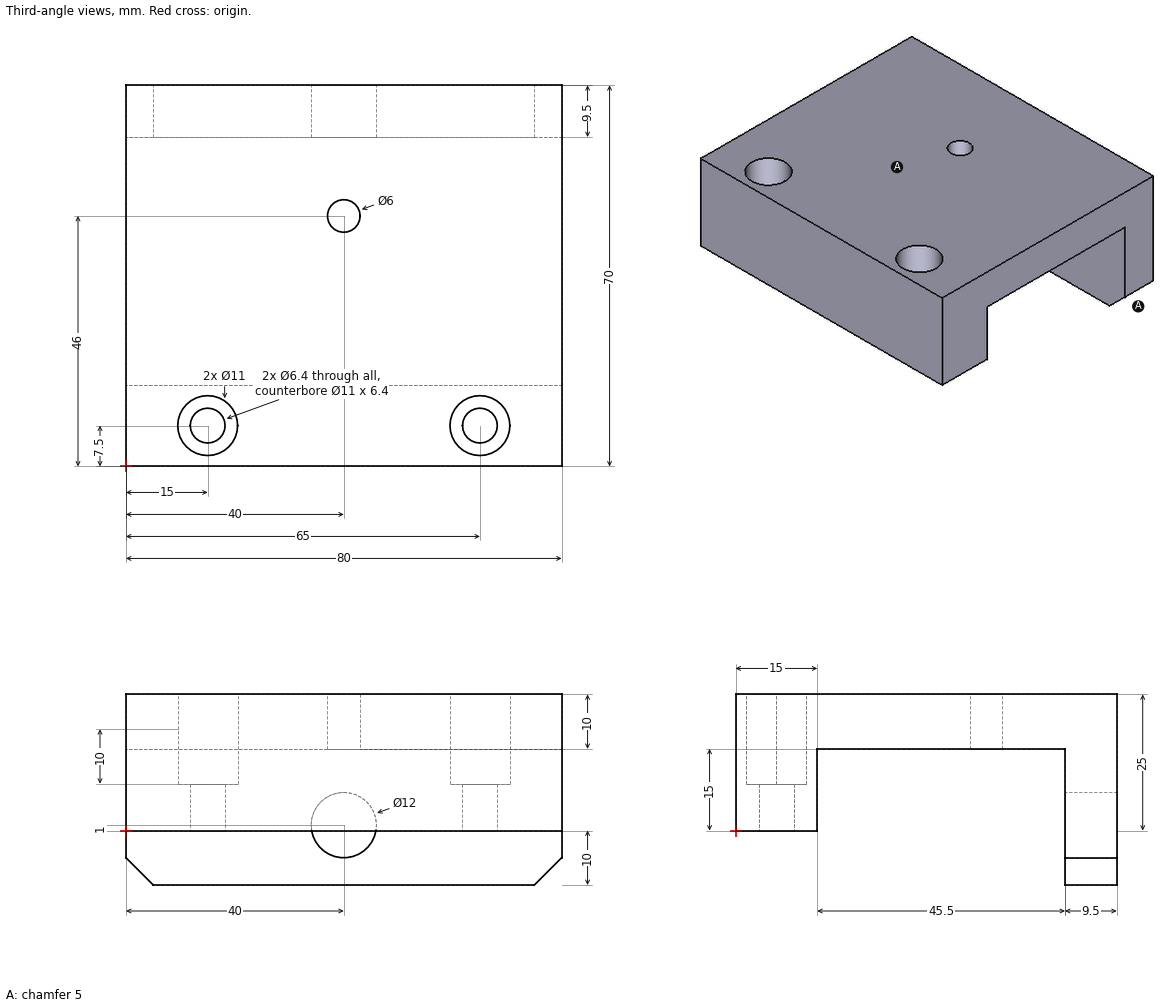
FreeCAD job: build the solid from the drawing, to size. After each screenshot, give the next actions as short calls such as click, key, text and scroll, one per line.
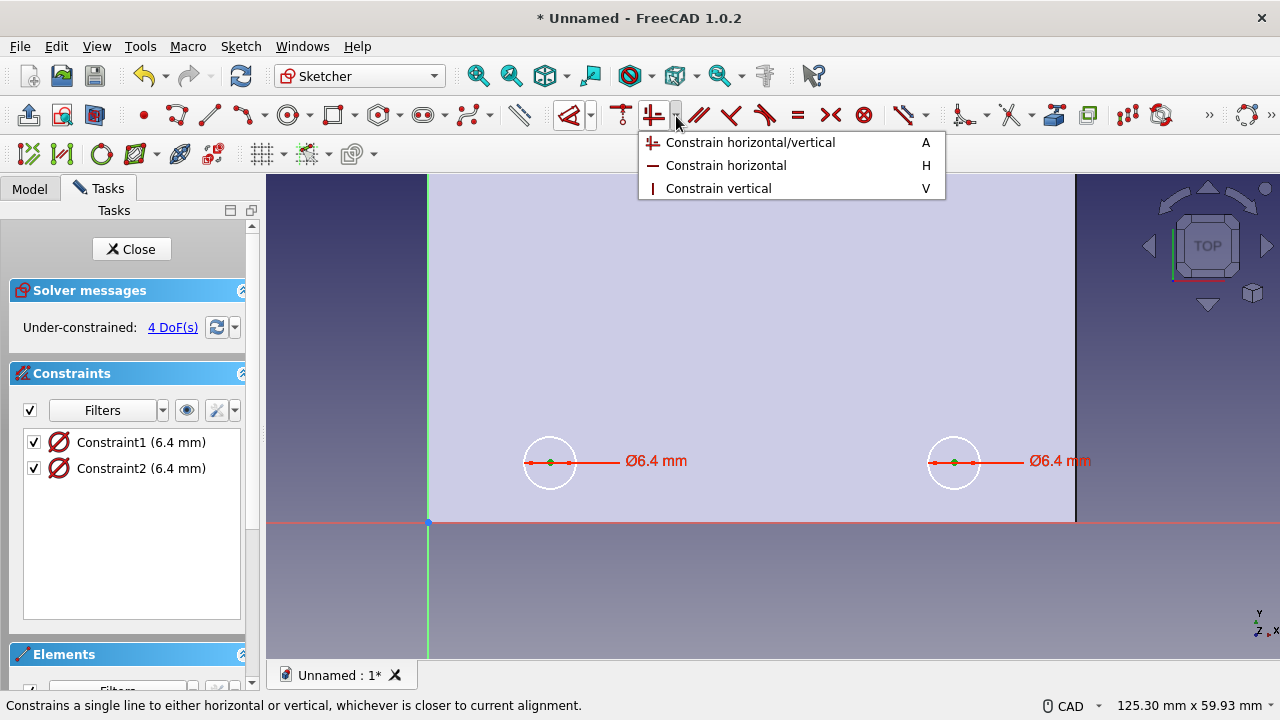
click(792, 166)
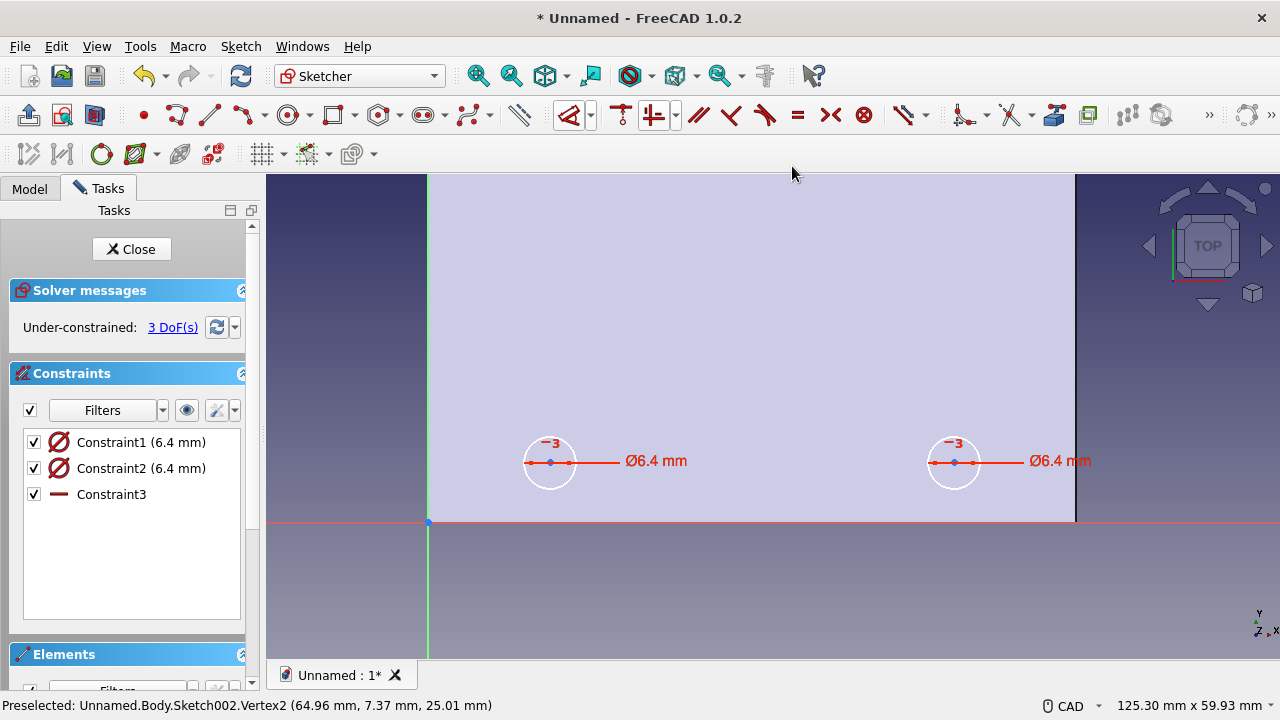
click(550, 463)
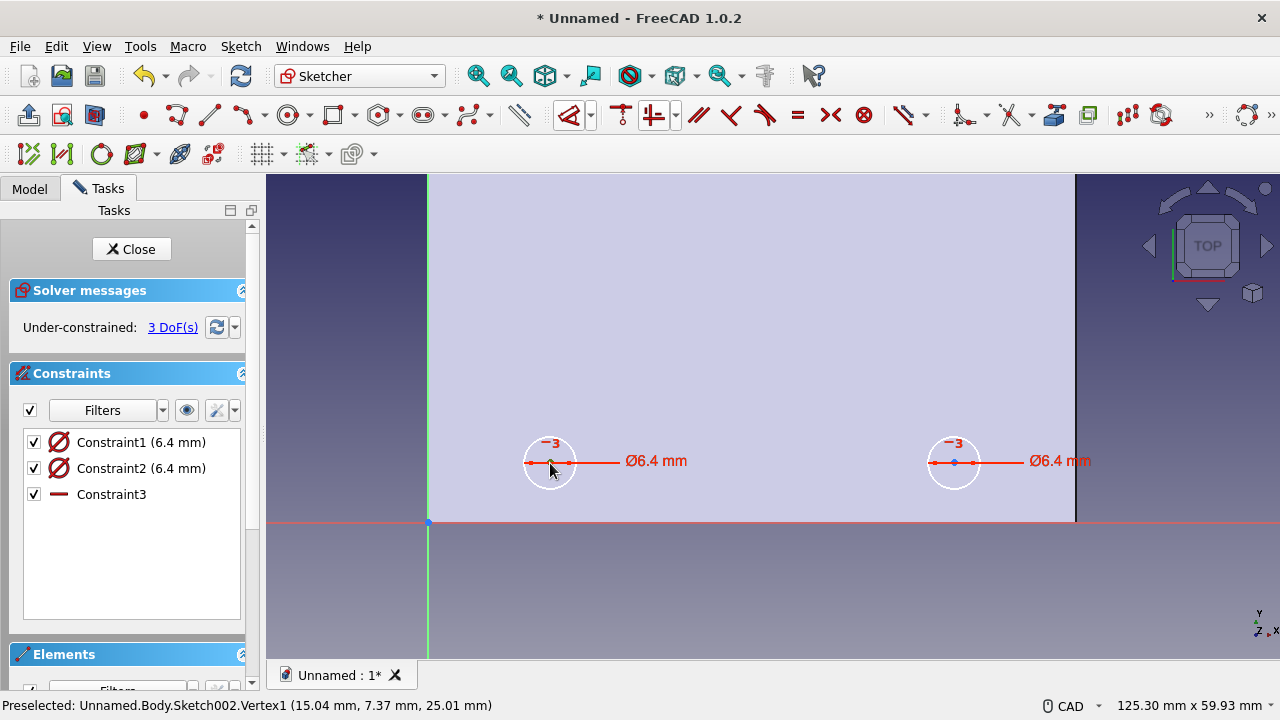
click(590, 116)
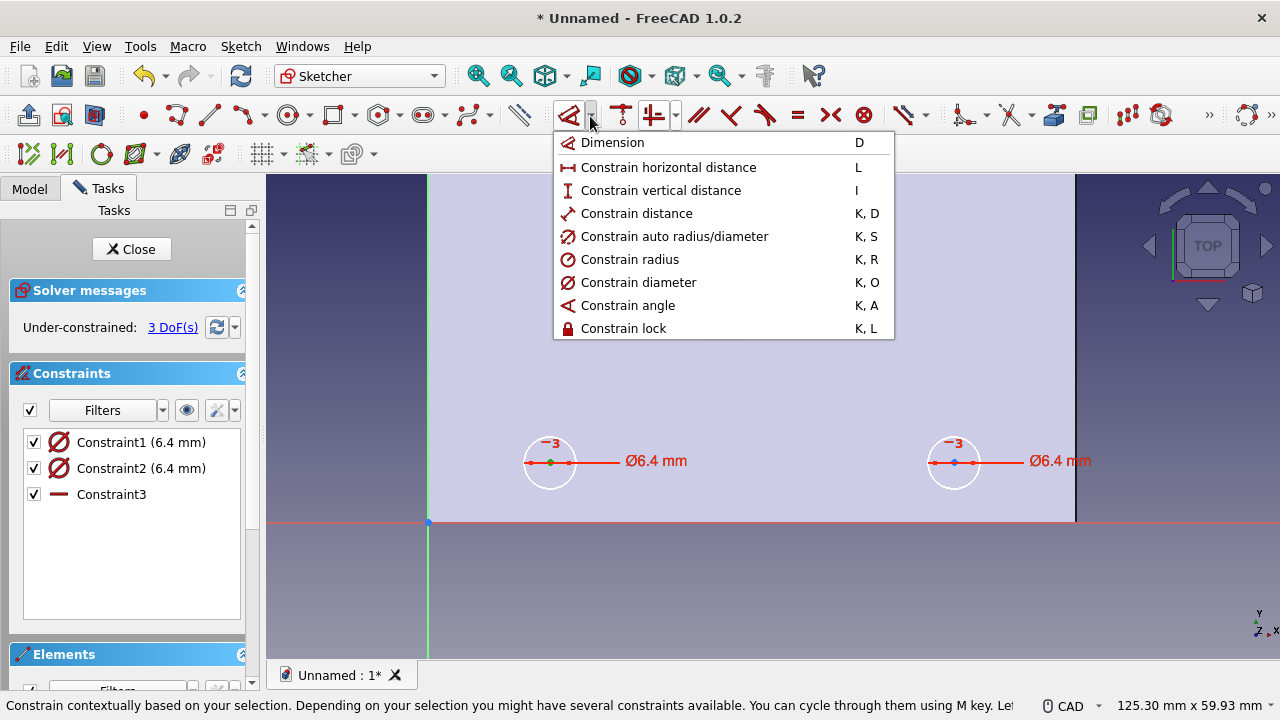
click(724, 168)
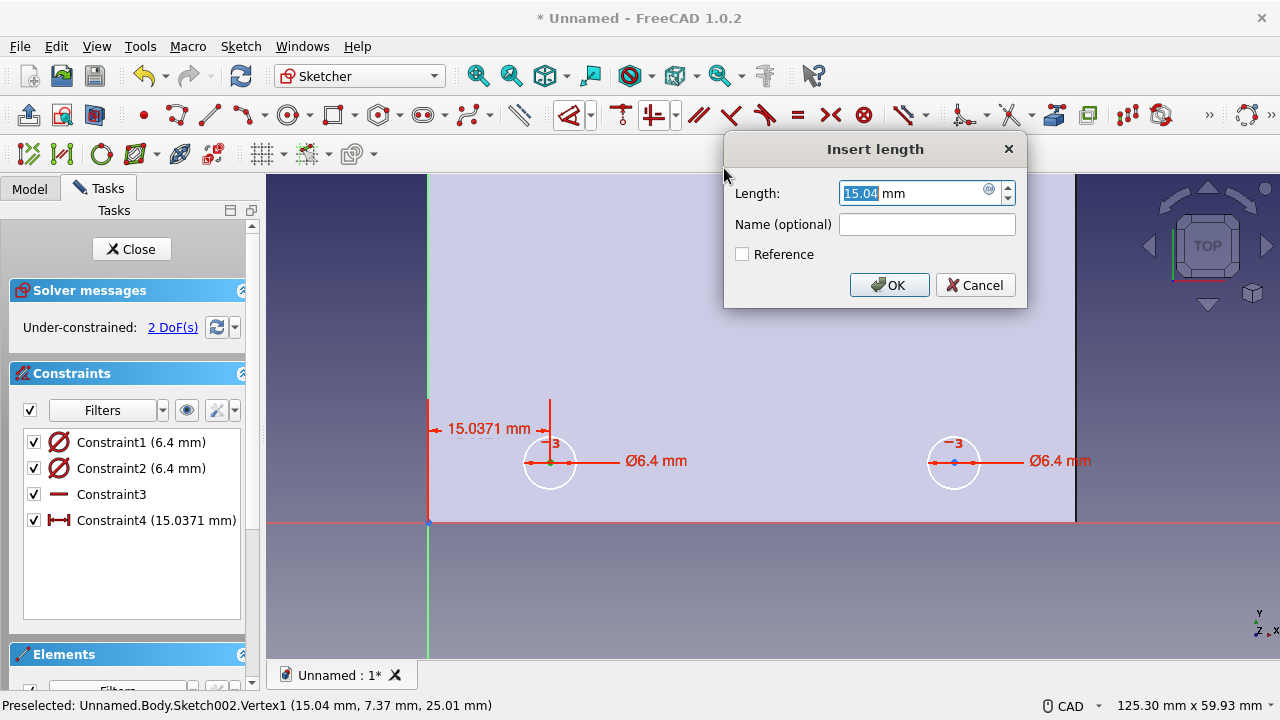
text(15)
key(Return)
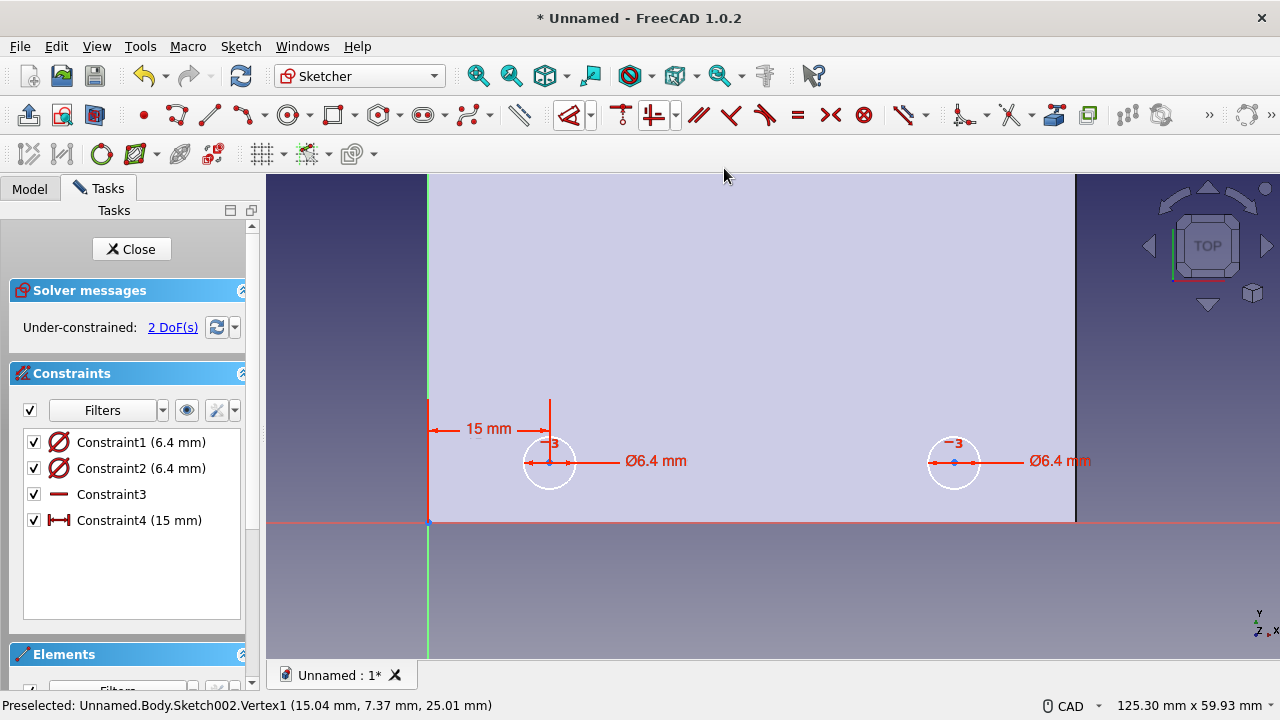
click(954, 463)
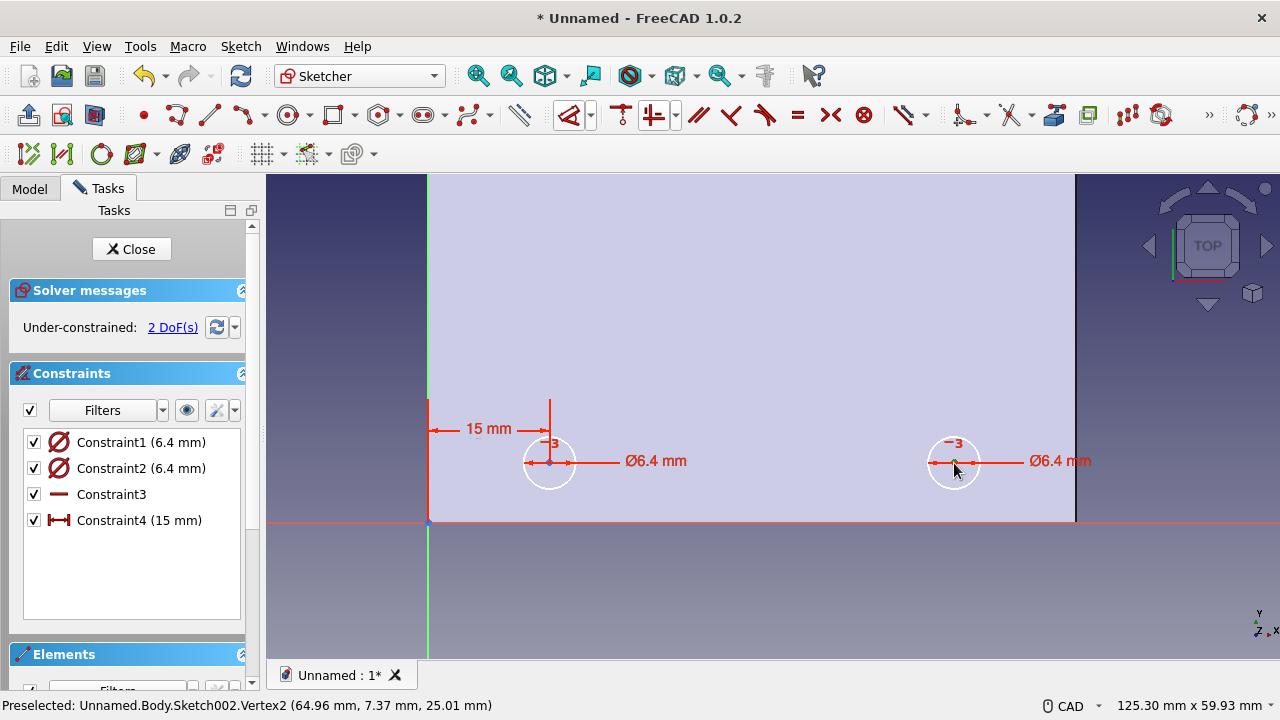
click(590, 116)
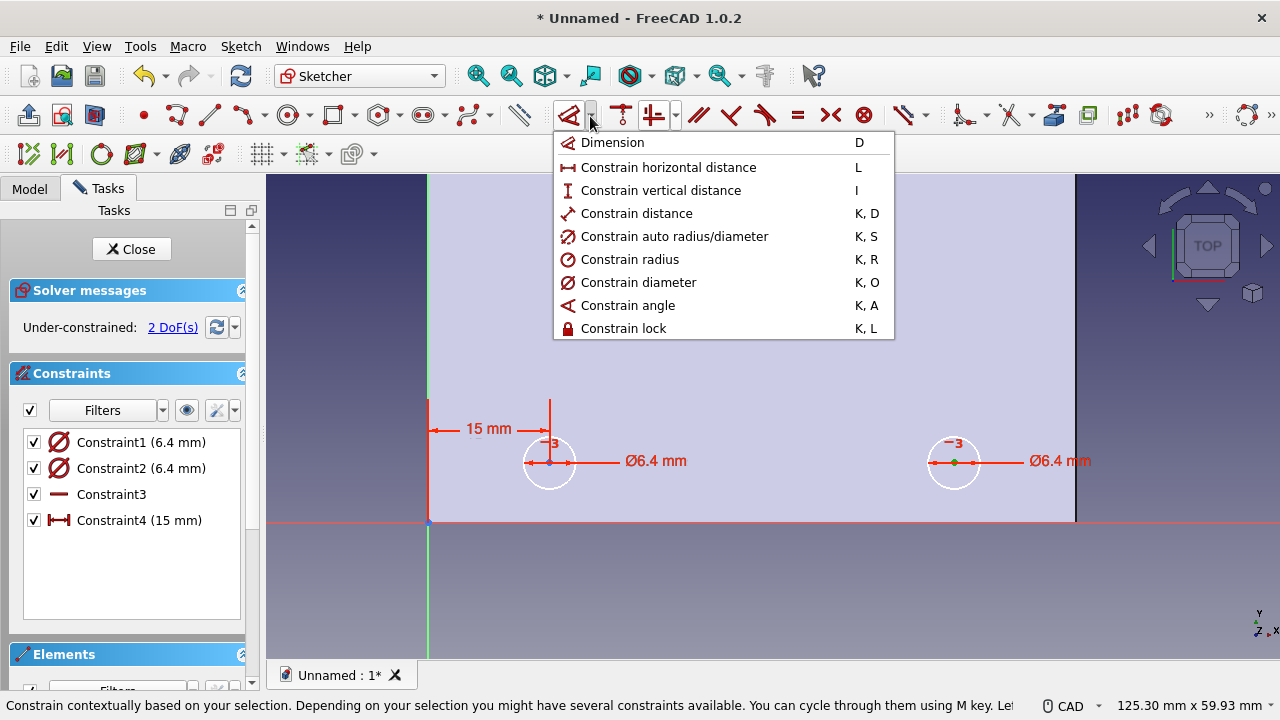
click(724, 168)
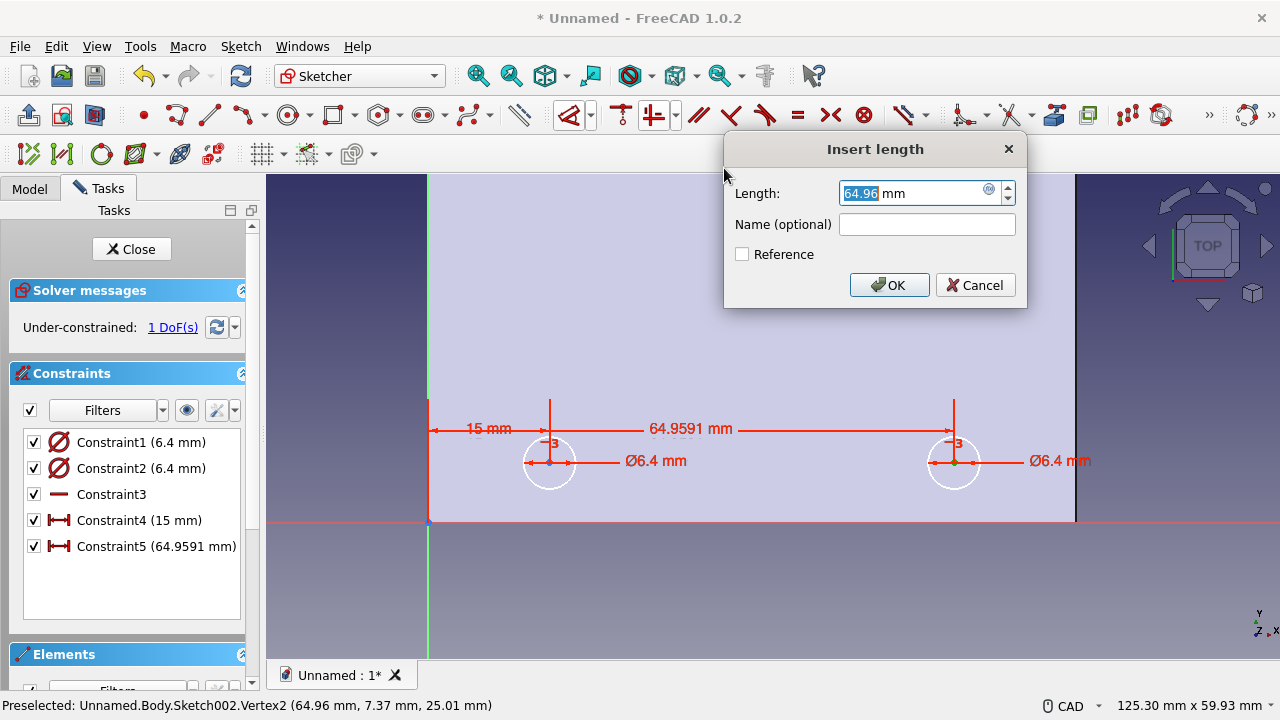
text(65)
key(Return)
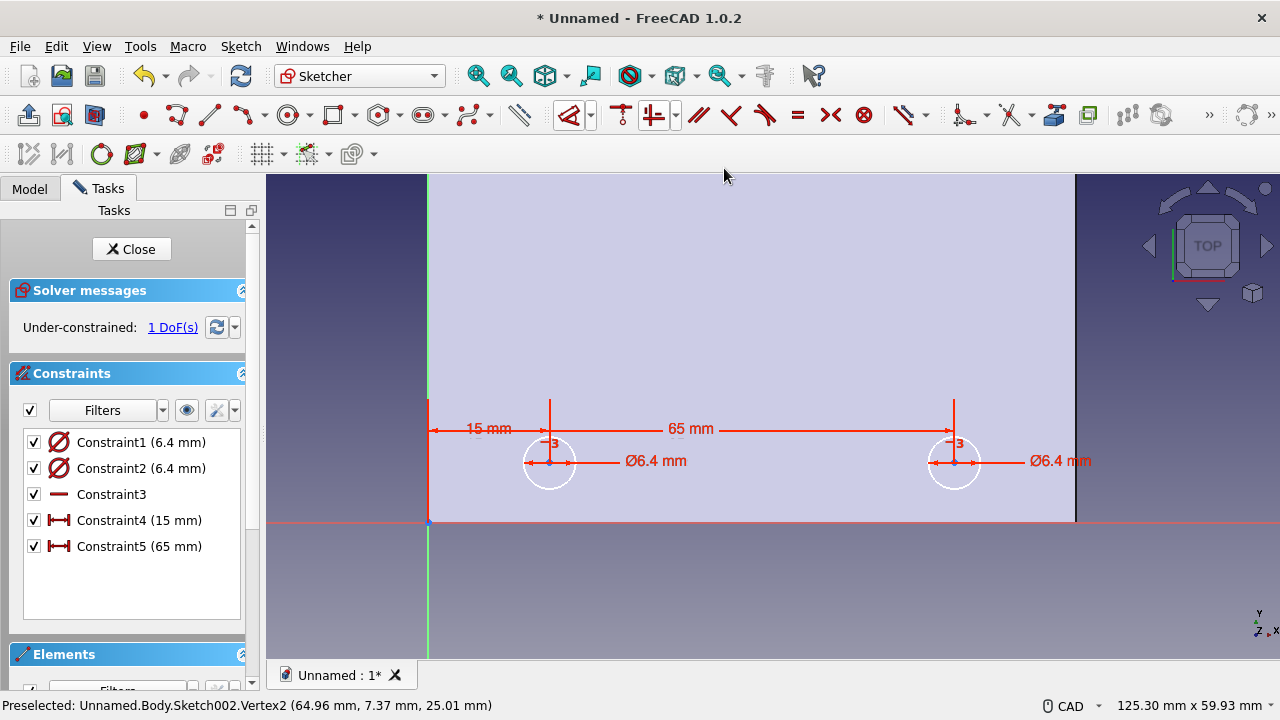
click(550, 463)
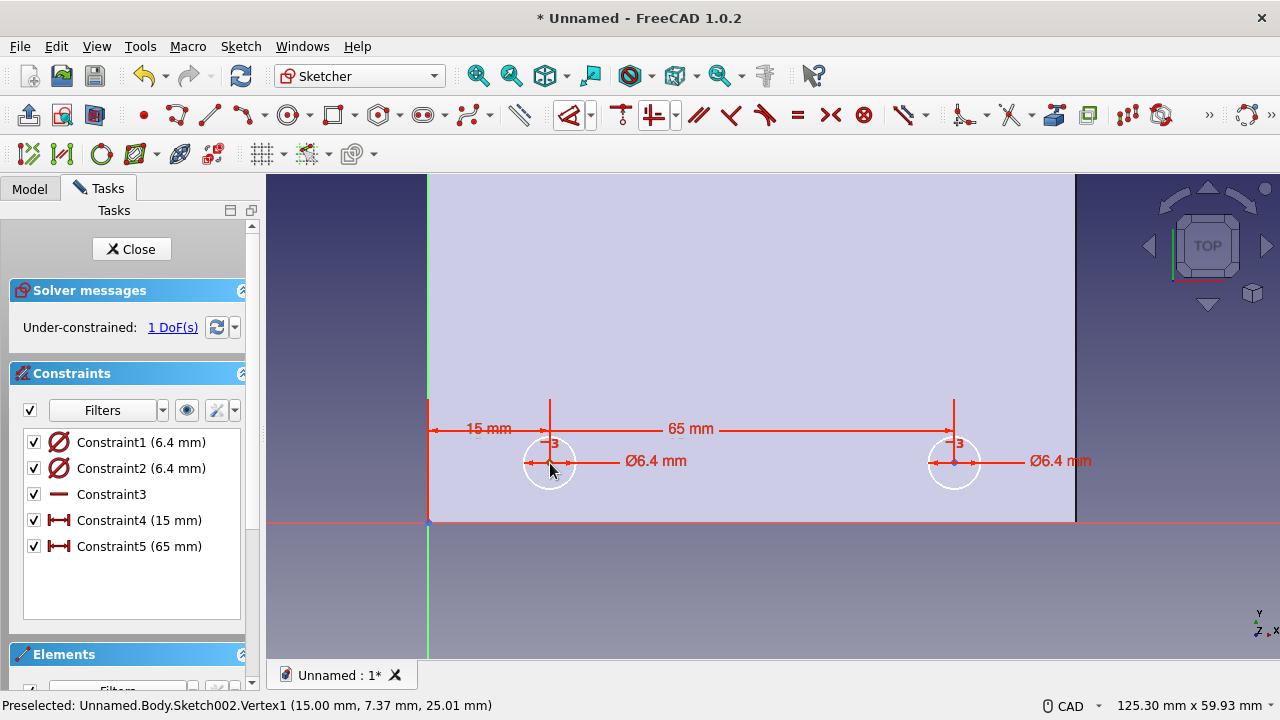
click(590, 116)